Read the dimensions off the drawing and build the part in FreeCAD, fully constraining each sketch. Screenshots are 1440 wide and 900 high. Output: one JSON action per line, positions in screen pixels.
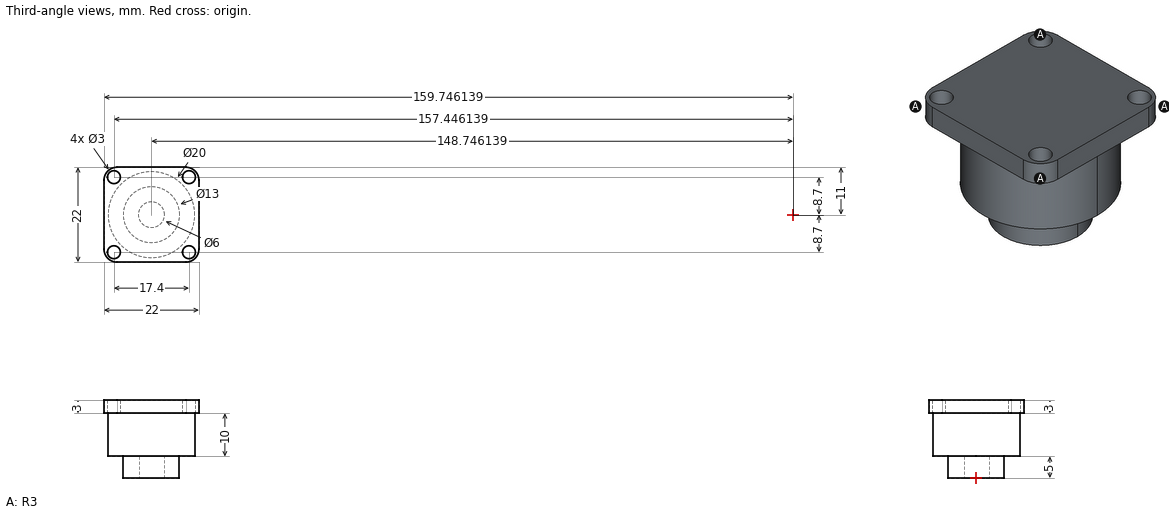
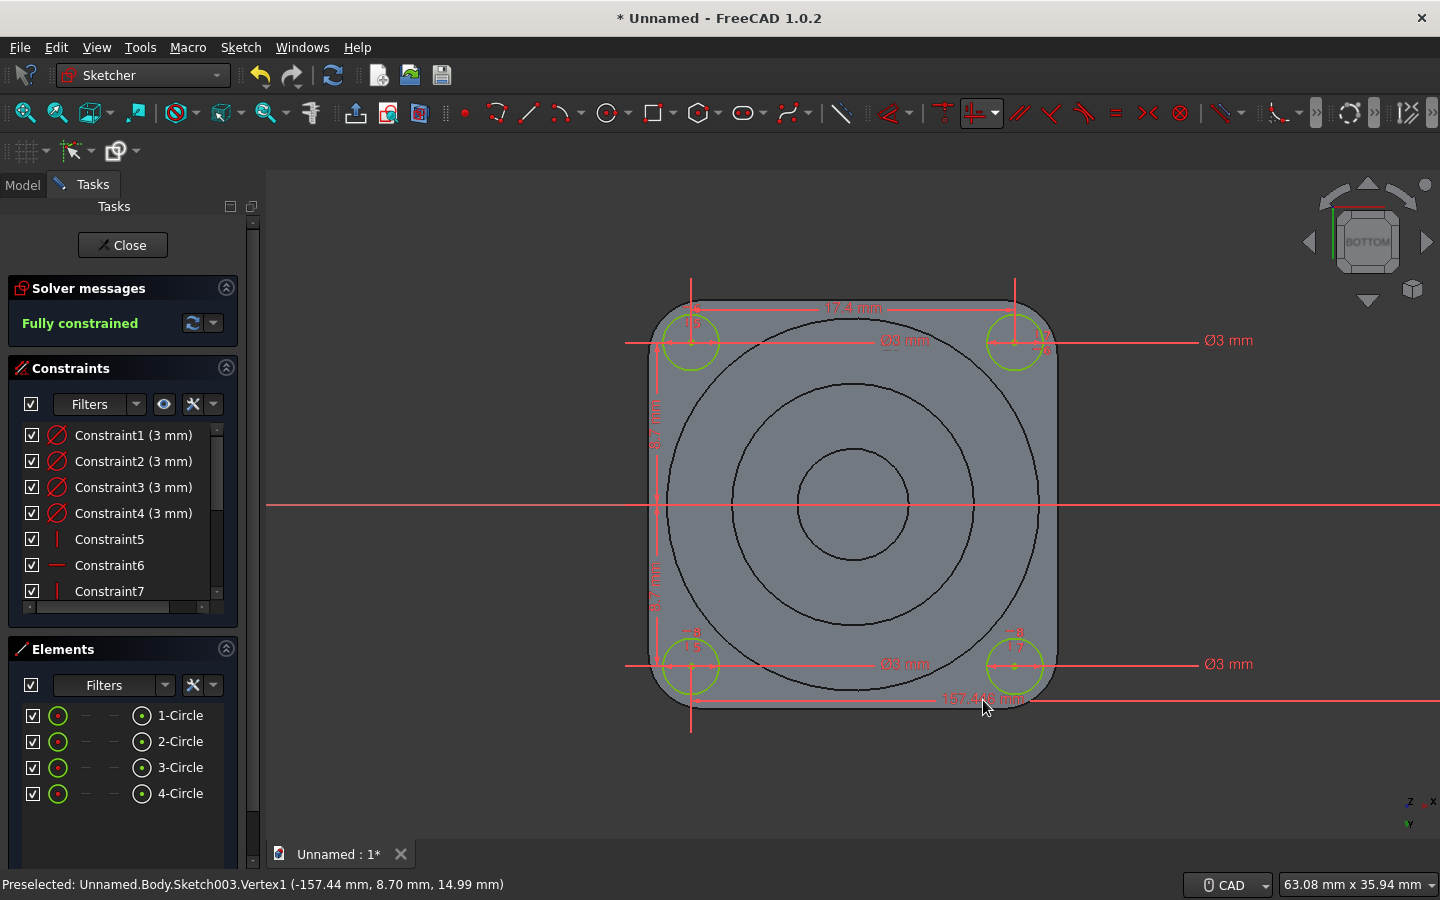
{"action": "left_click", "coordinate": [123, 245]}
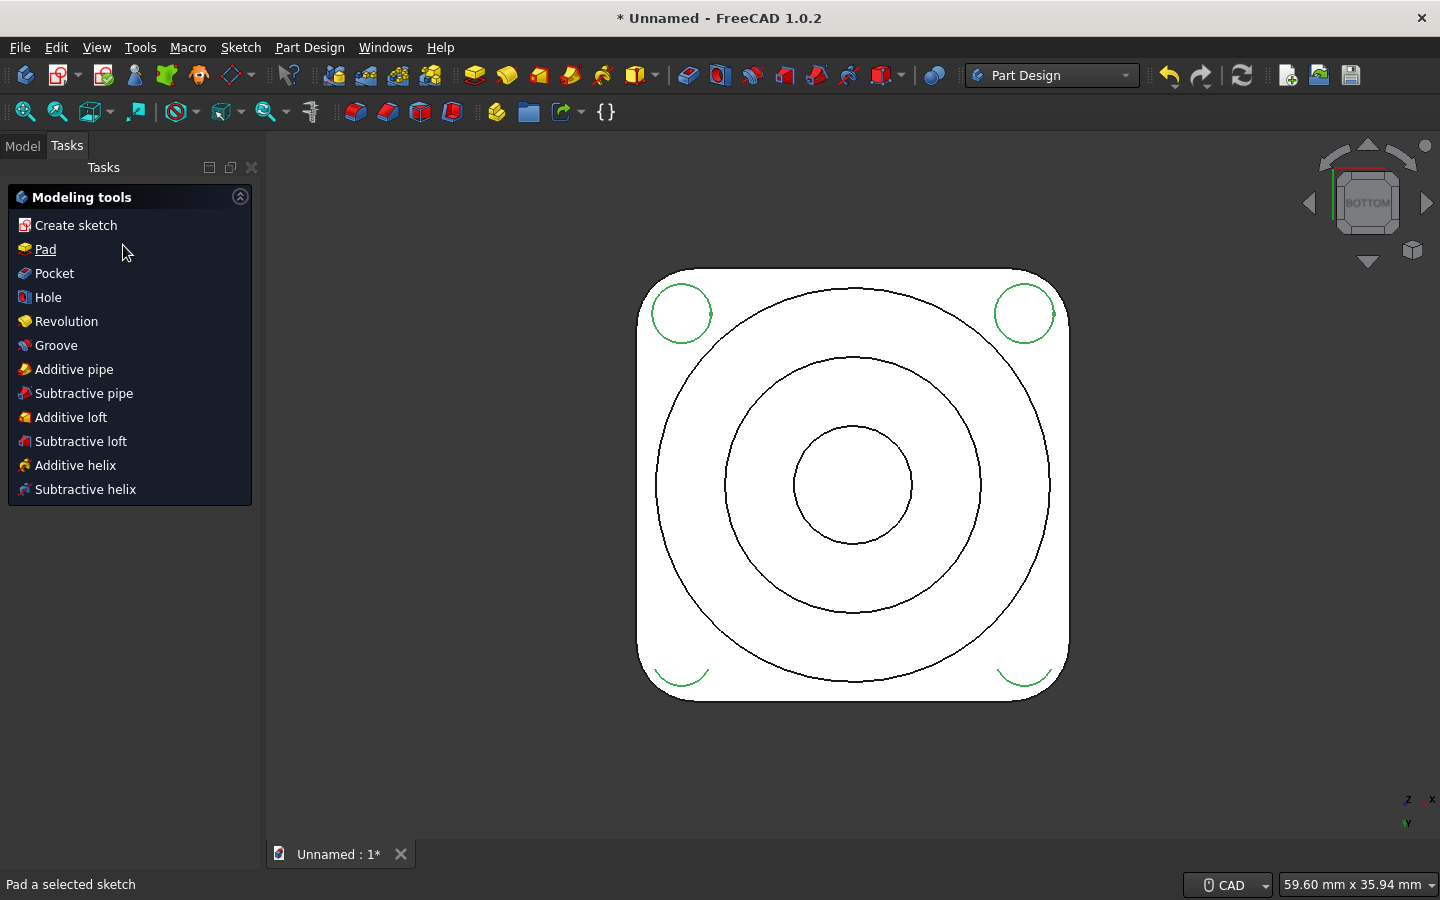
{"action": "left_click", "coordinate": [690, 76]}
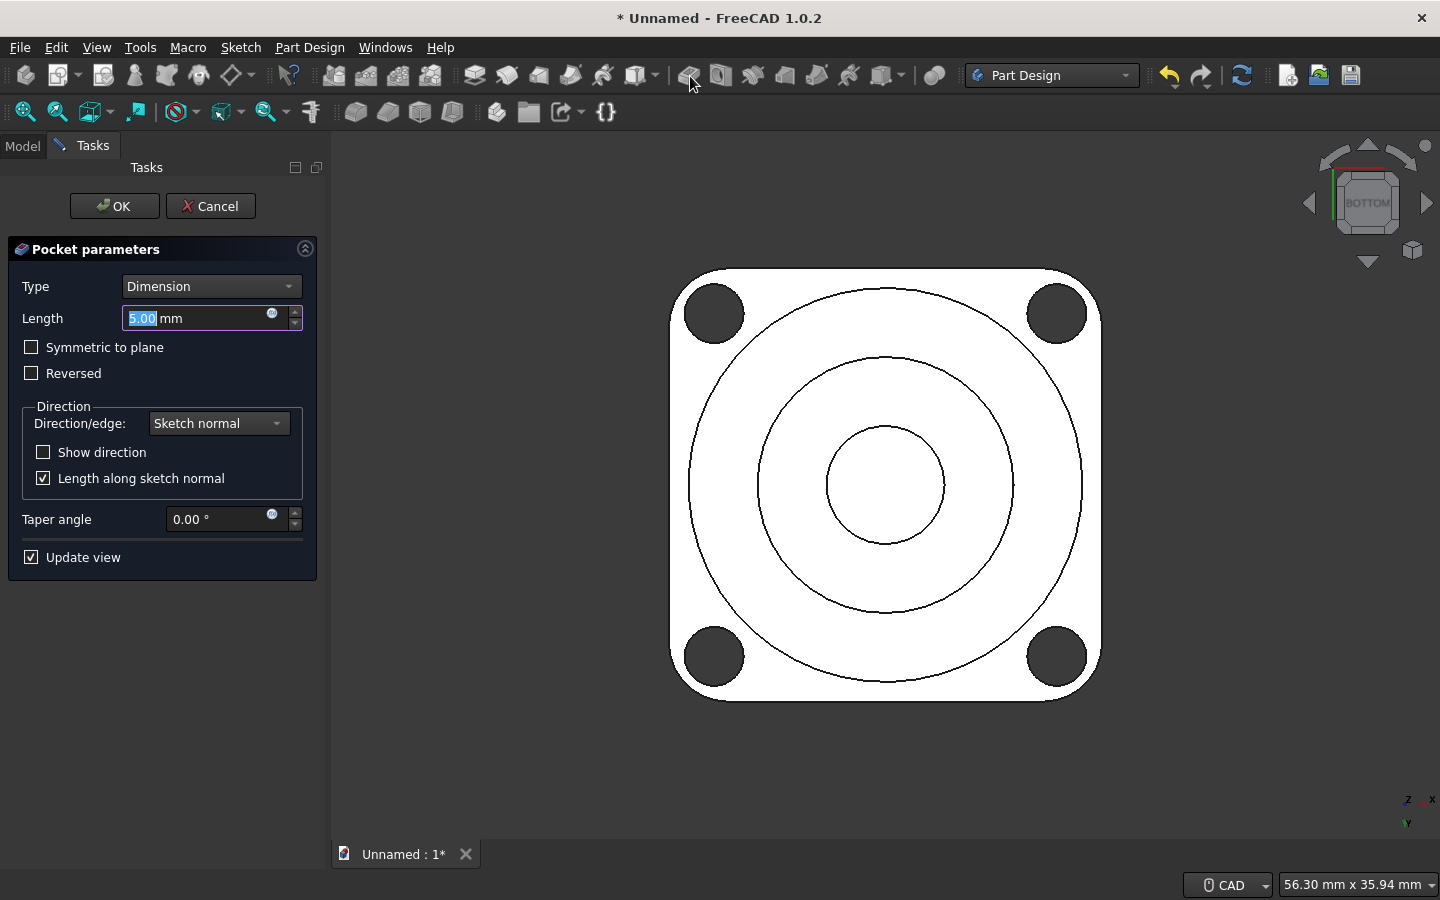
{"action": "type", "text": "3"}
{"action": "key", "text": "Tab"}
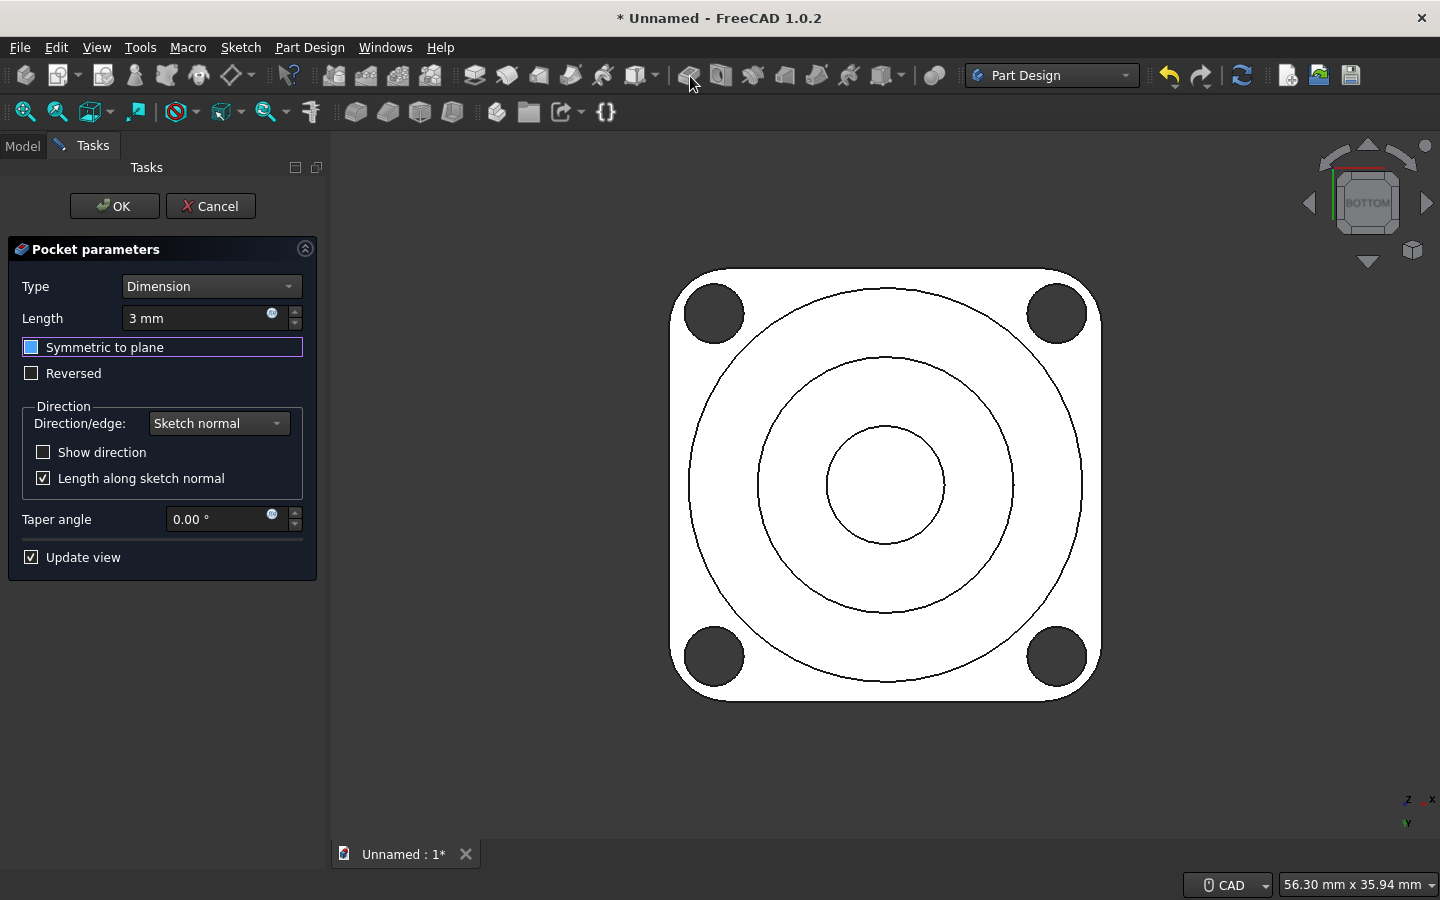
{"action": "left_click", "coordinate": [115, 206]}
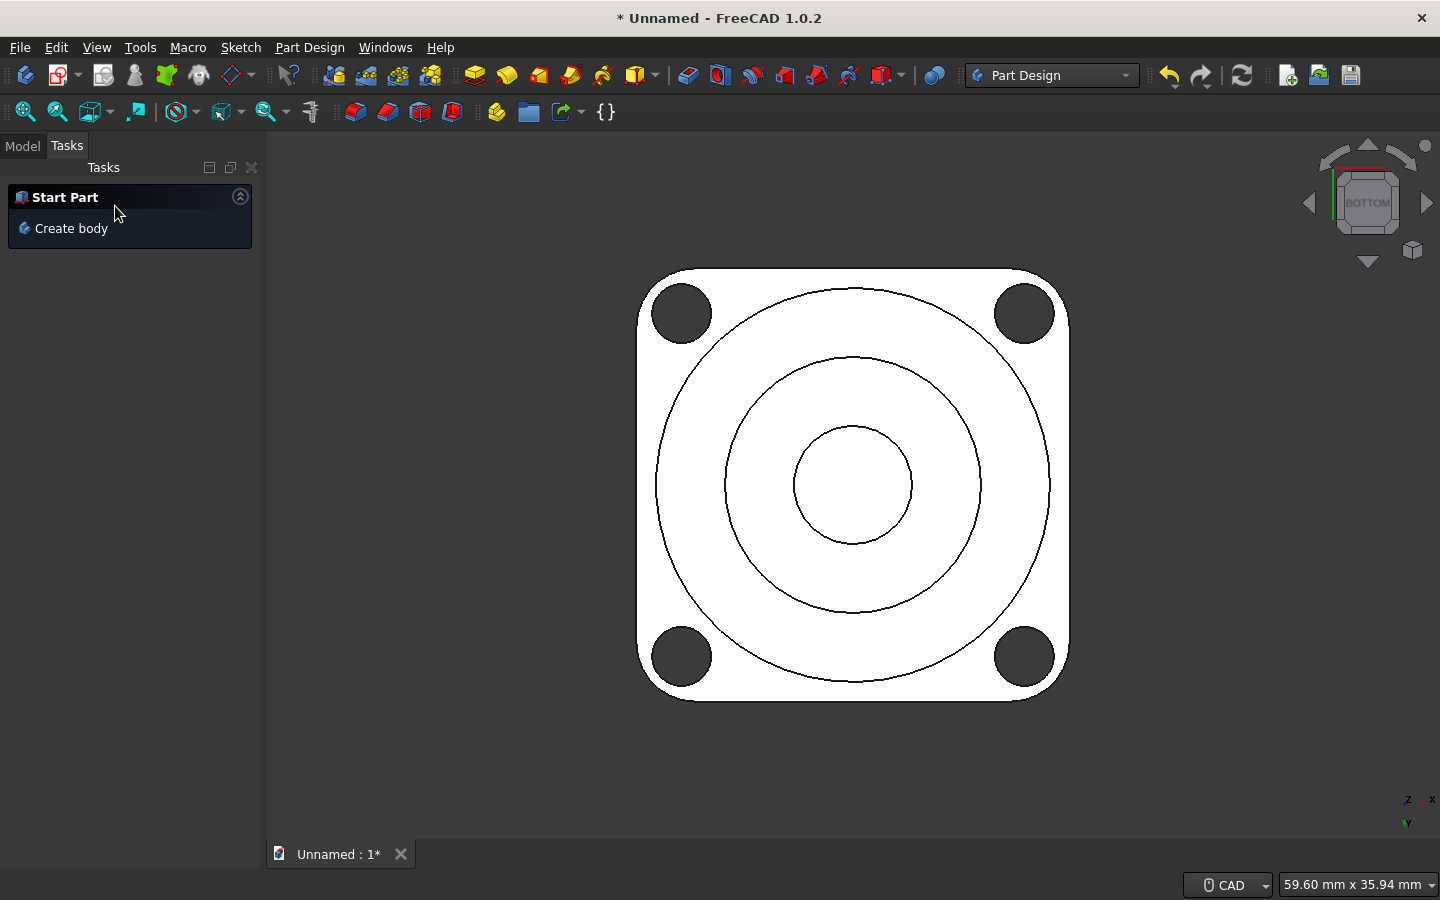
{"action": "key", "text": "0"}